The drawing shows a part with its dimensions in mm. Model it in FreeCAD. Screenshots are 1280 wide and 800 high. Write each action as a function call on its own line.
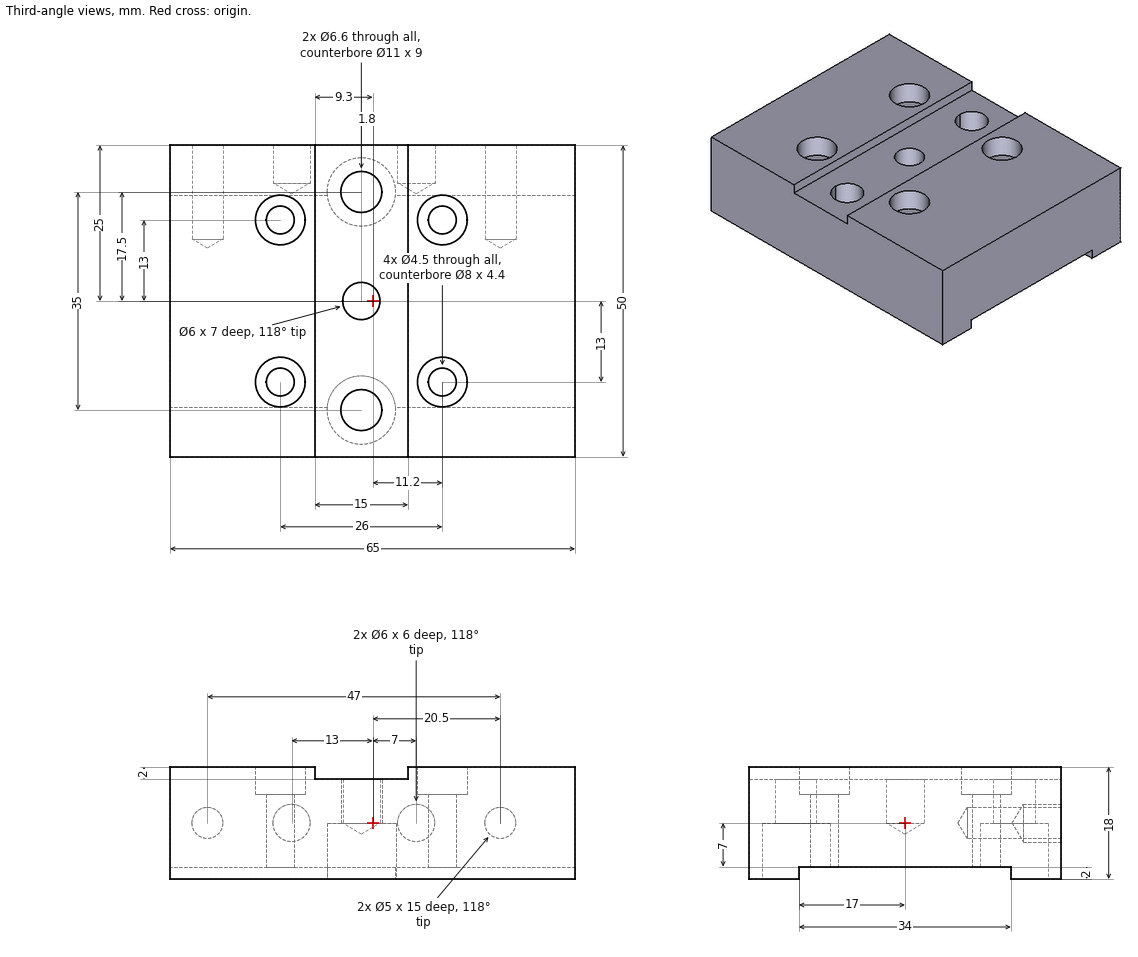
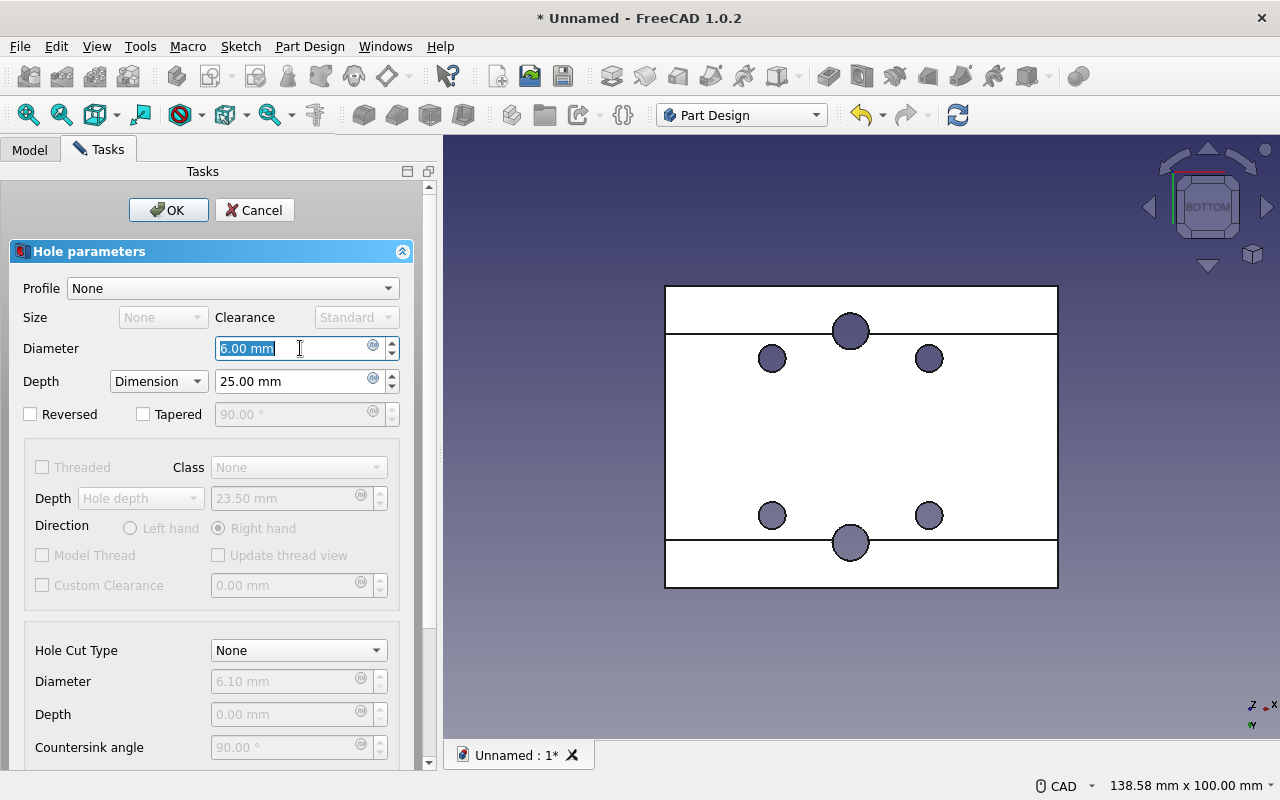
text(6.6)
key(Tab)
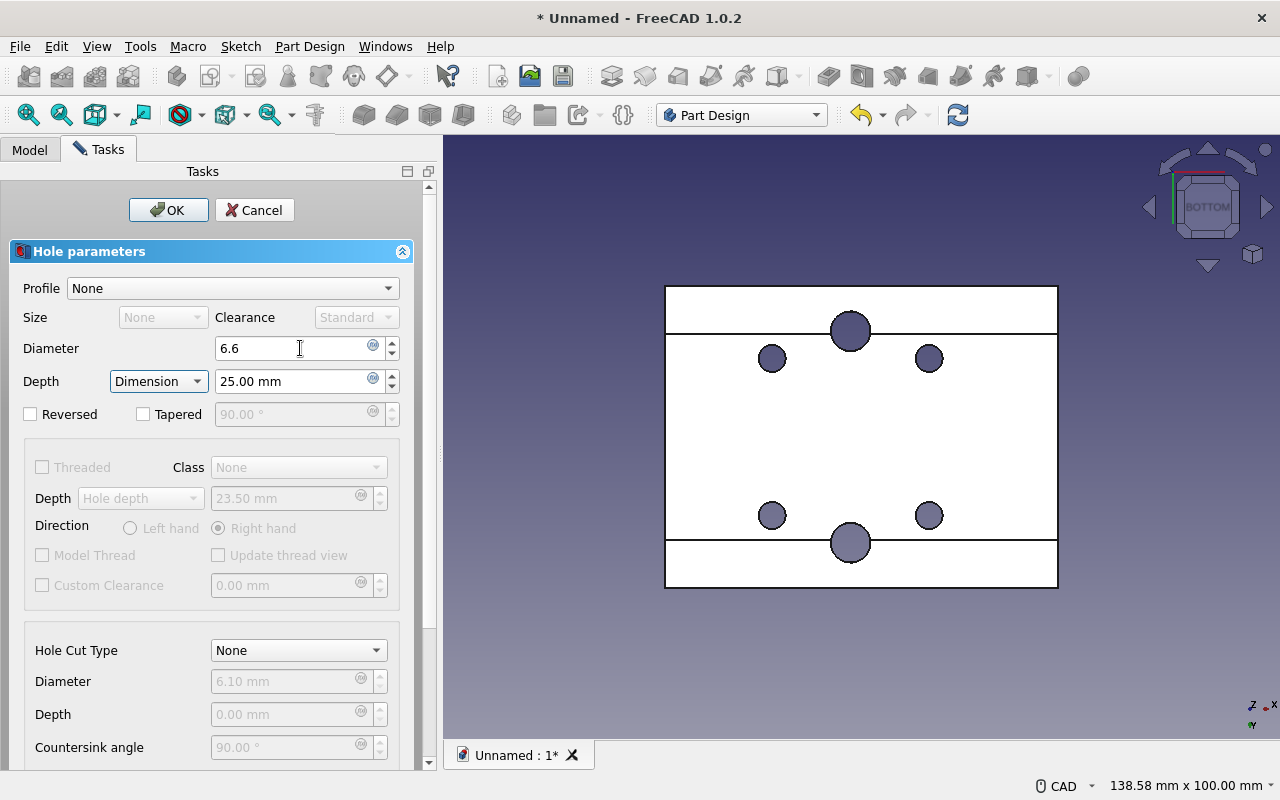
click(160, 382)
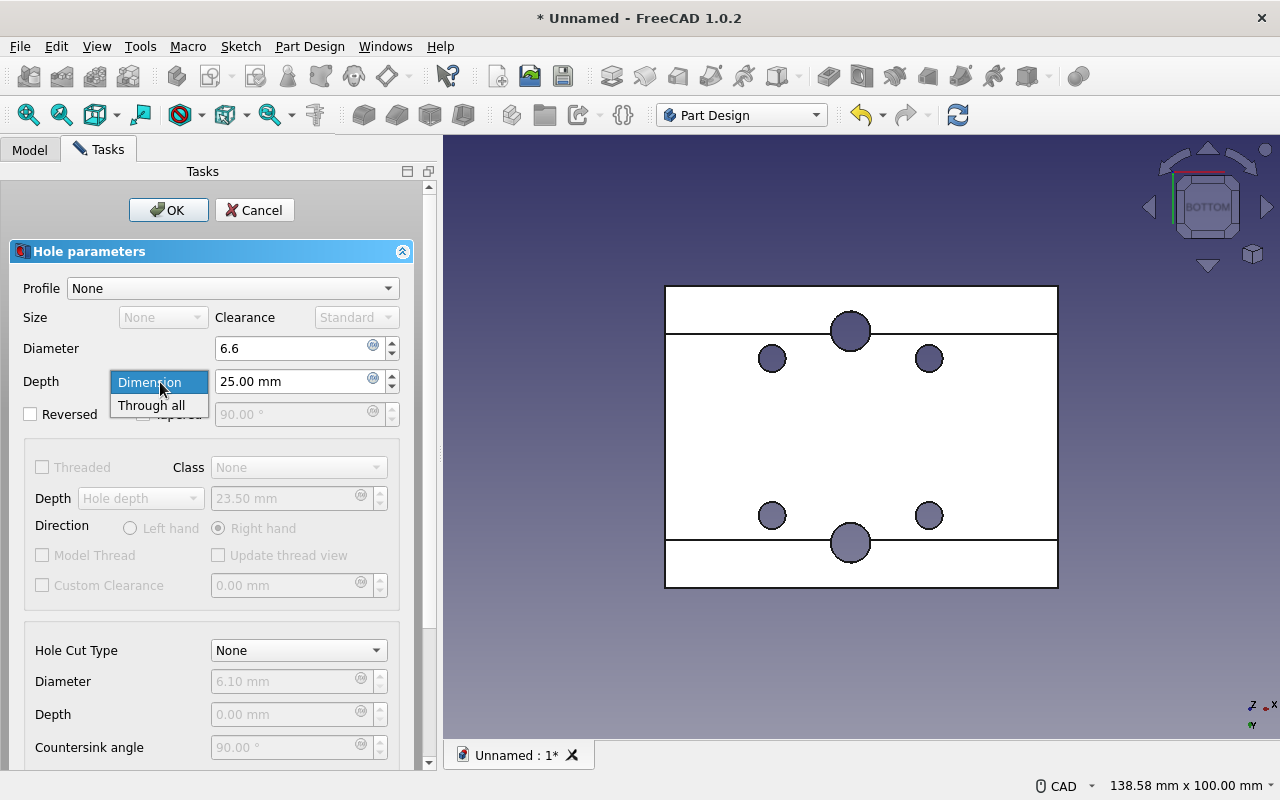
click(158, 406)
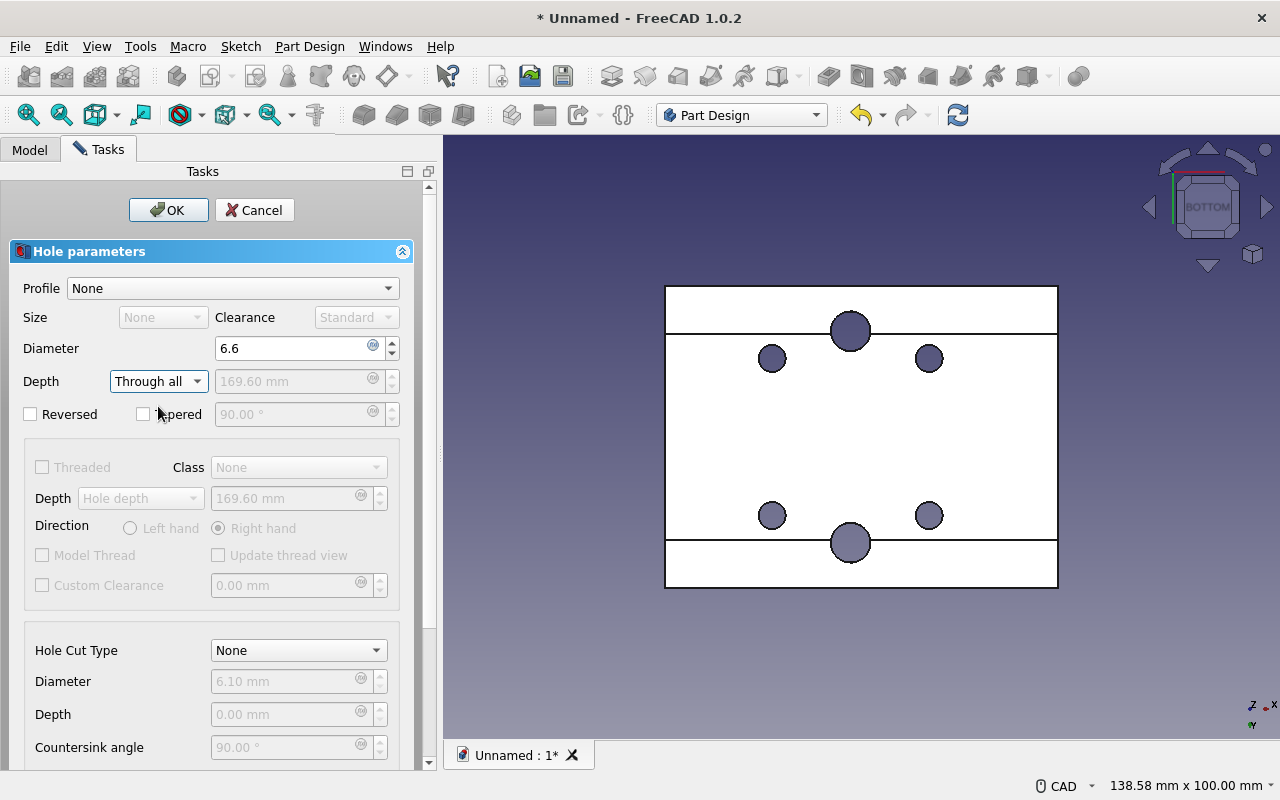
click(300, 650)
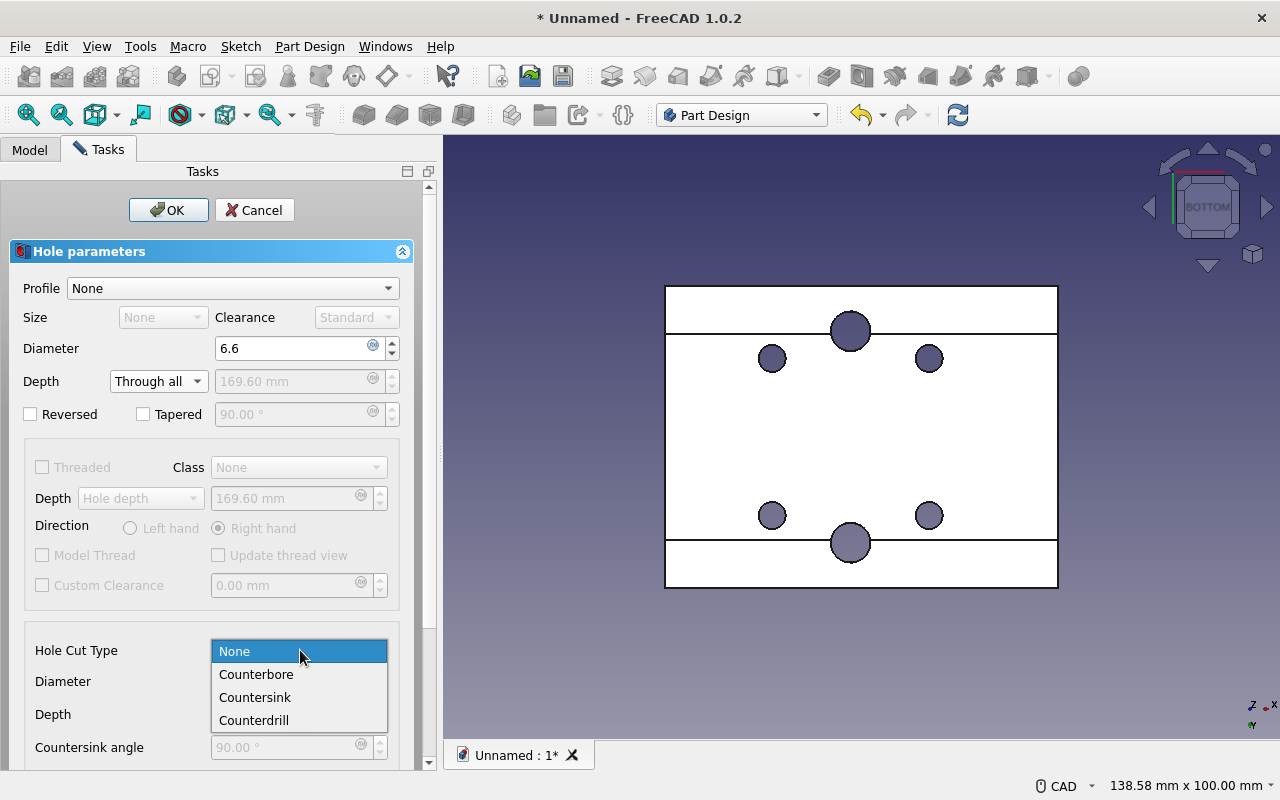
click(298, 674)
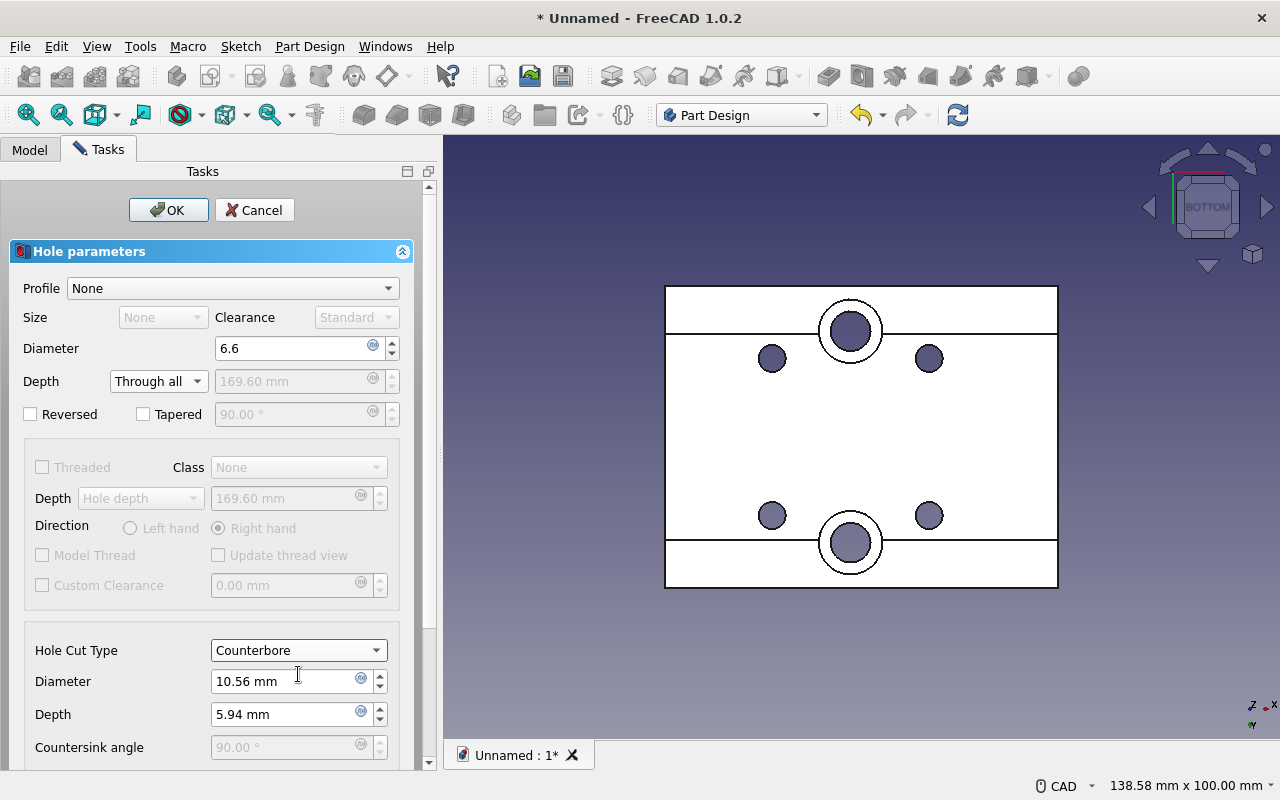
triple_click(292, 682)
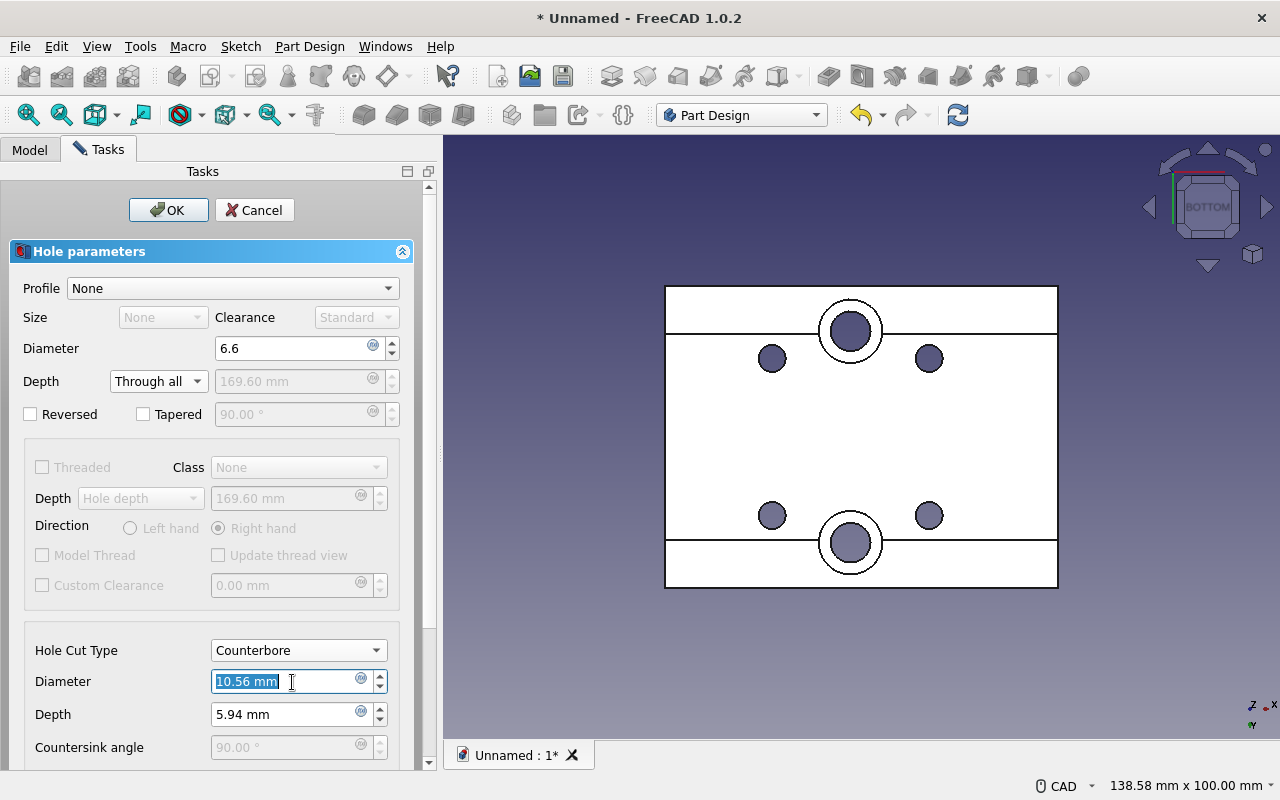
text(11)
key(Tab)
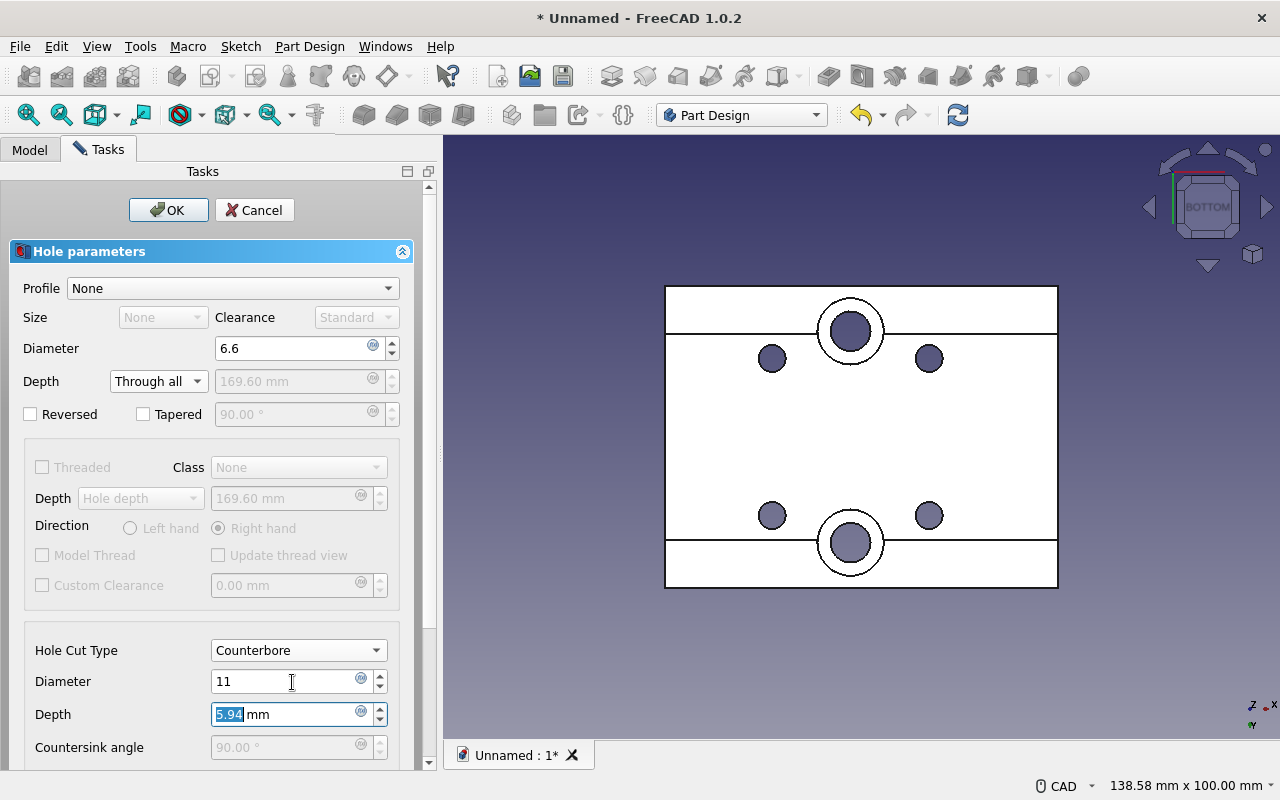
text(9)
key(Tab)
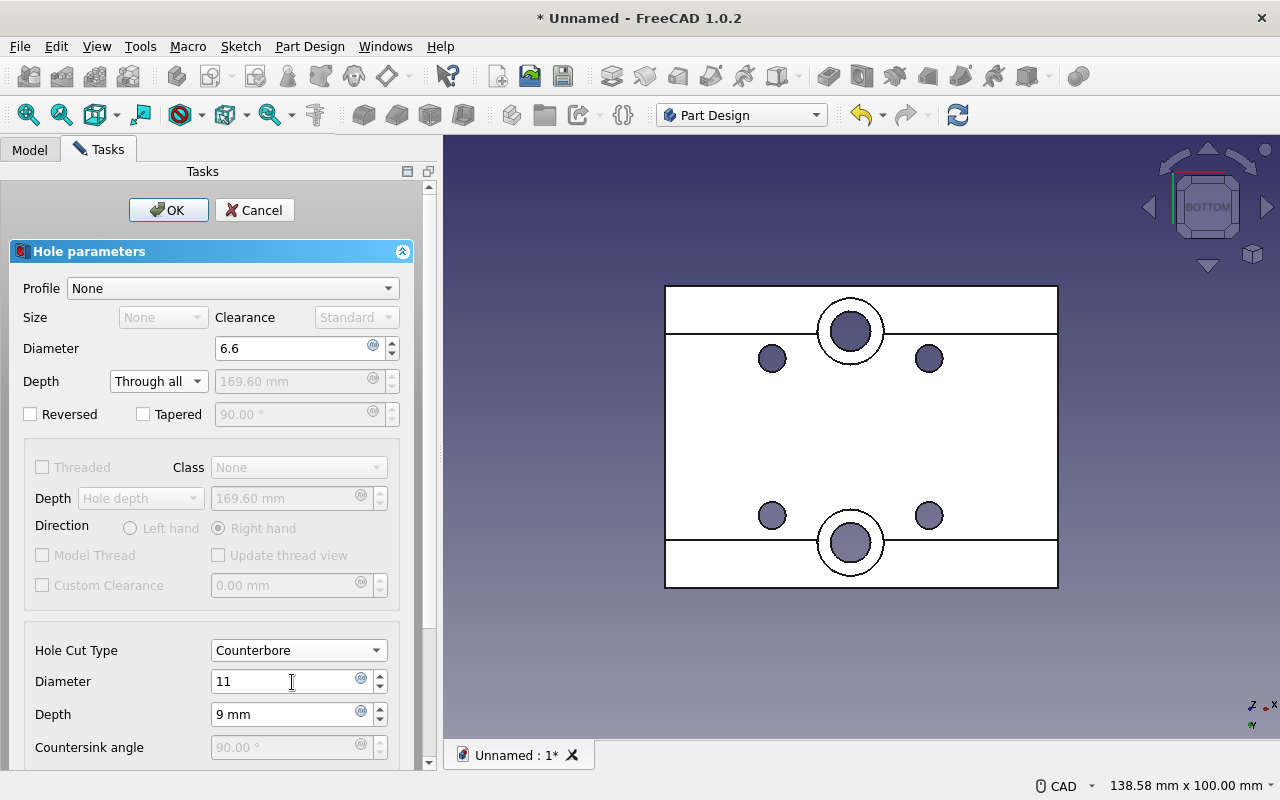
click(169, 210)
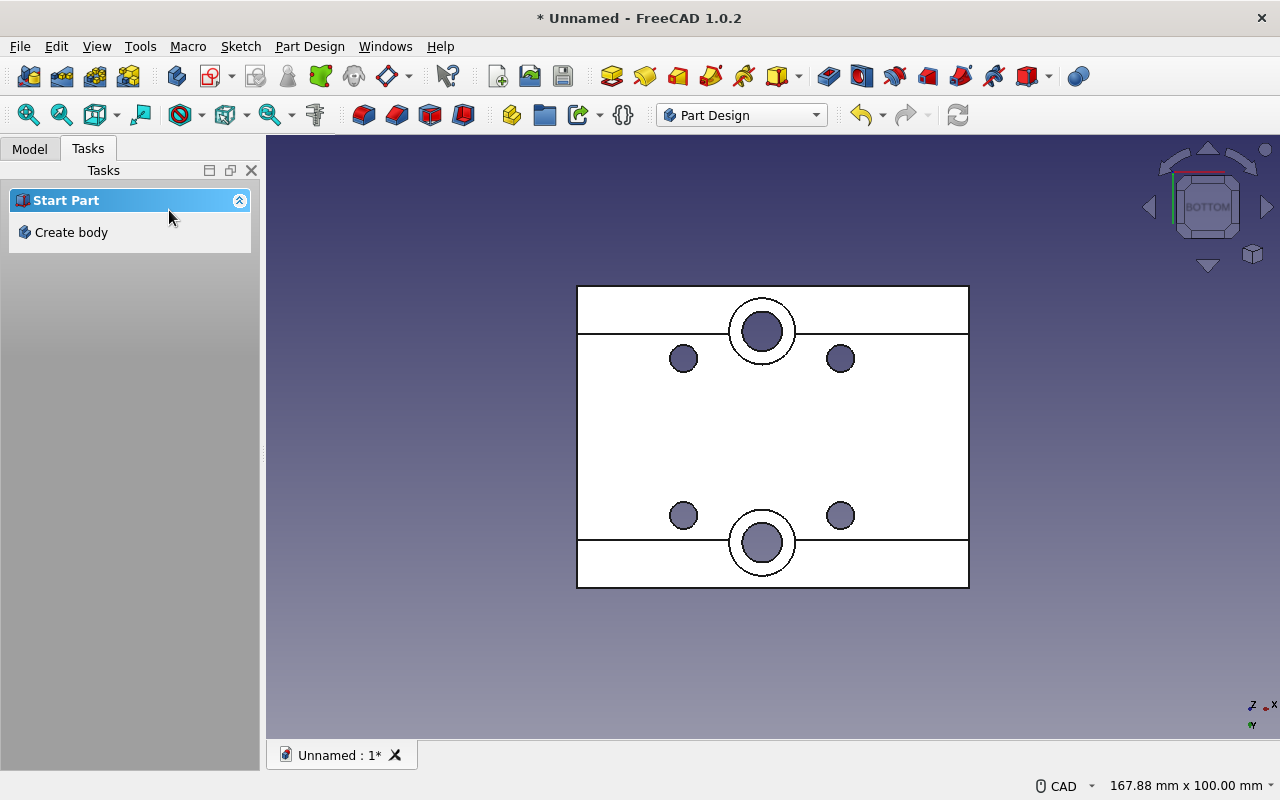
key(4)